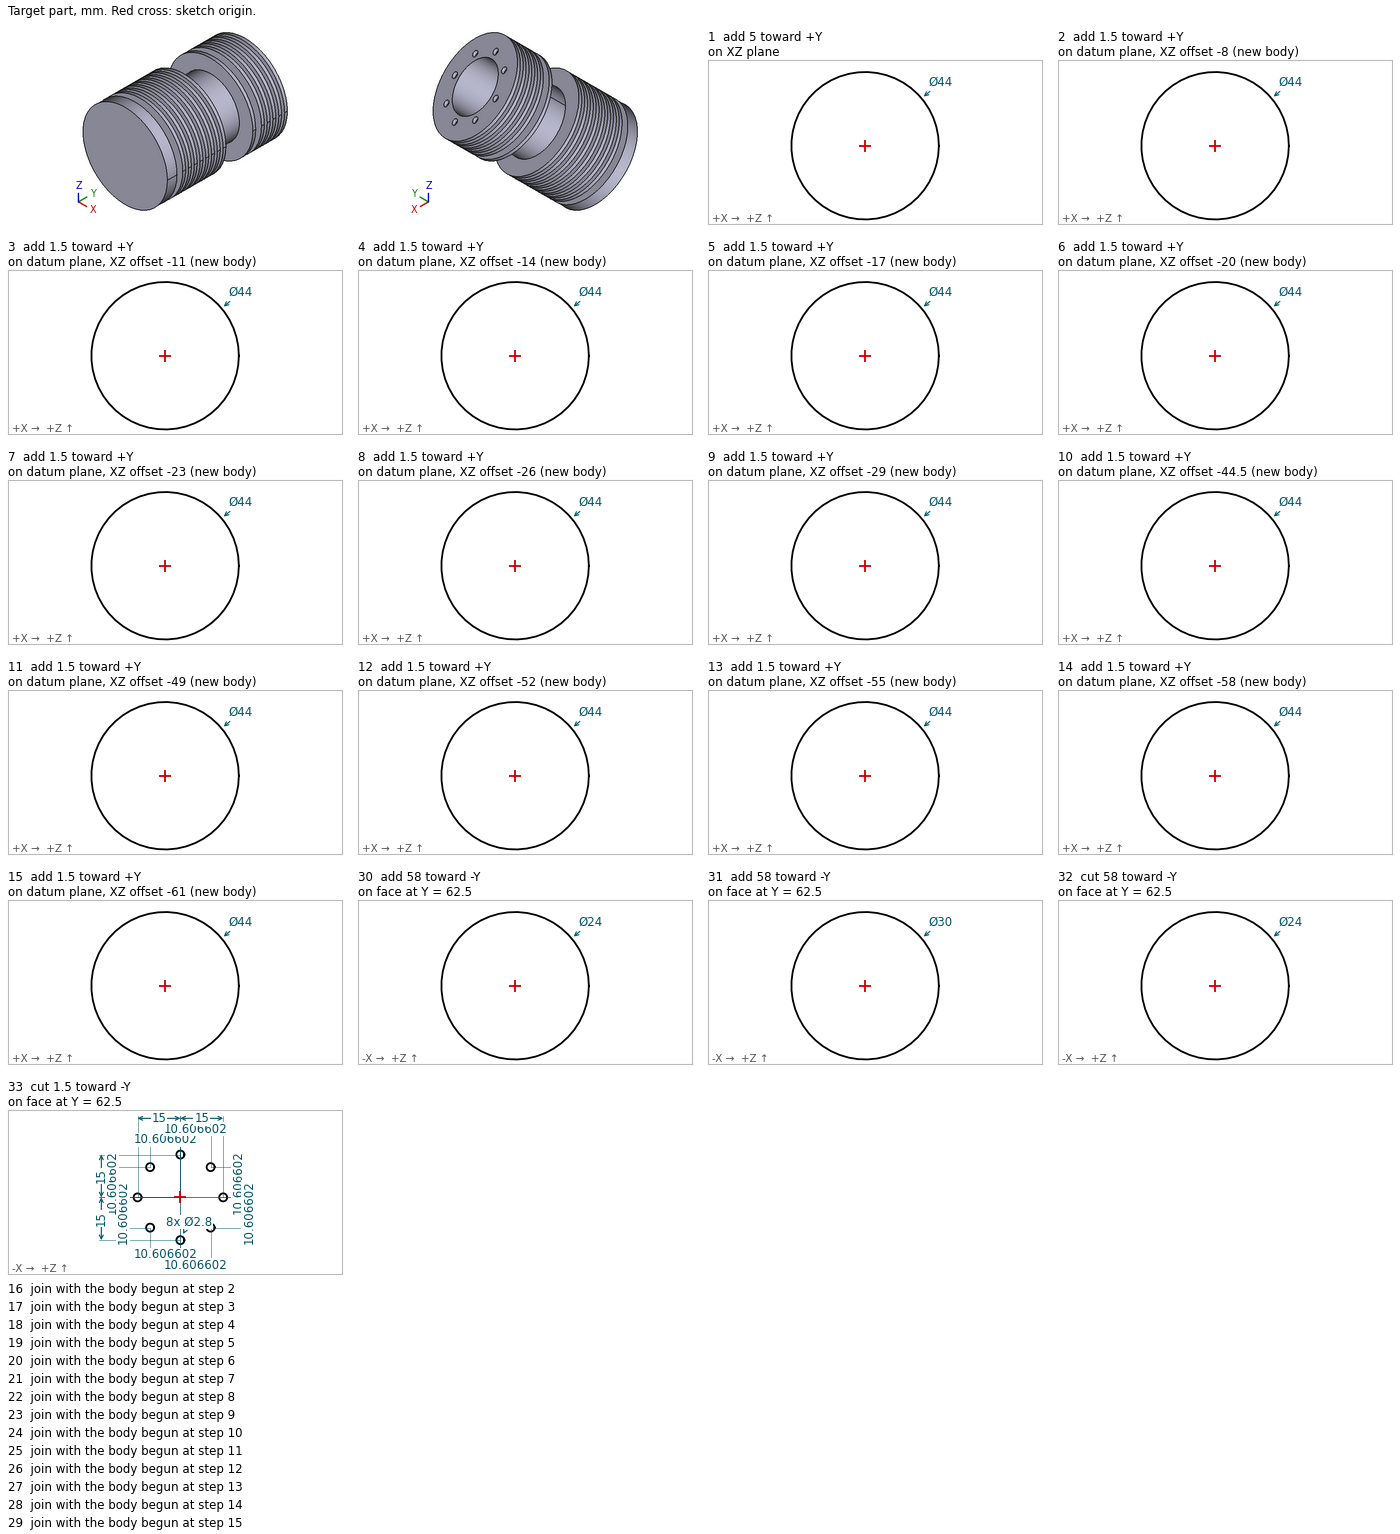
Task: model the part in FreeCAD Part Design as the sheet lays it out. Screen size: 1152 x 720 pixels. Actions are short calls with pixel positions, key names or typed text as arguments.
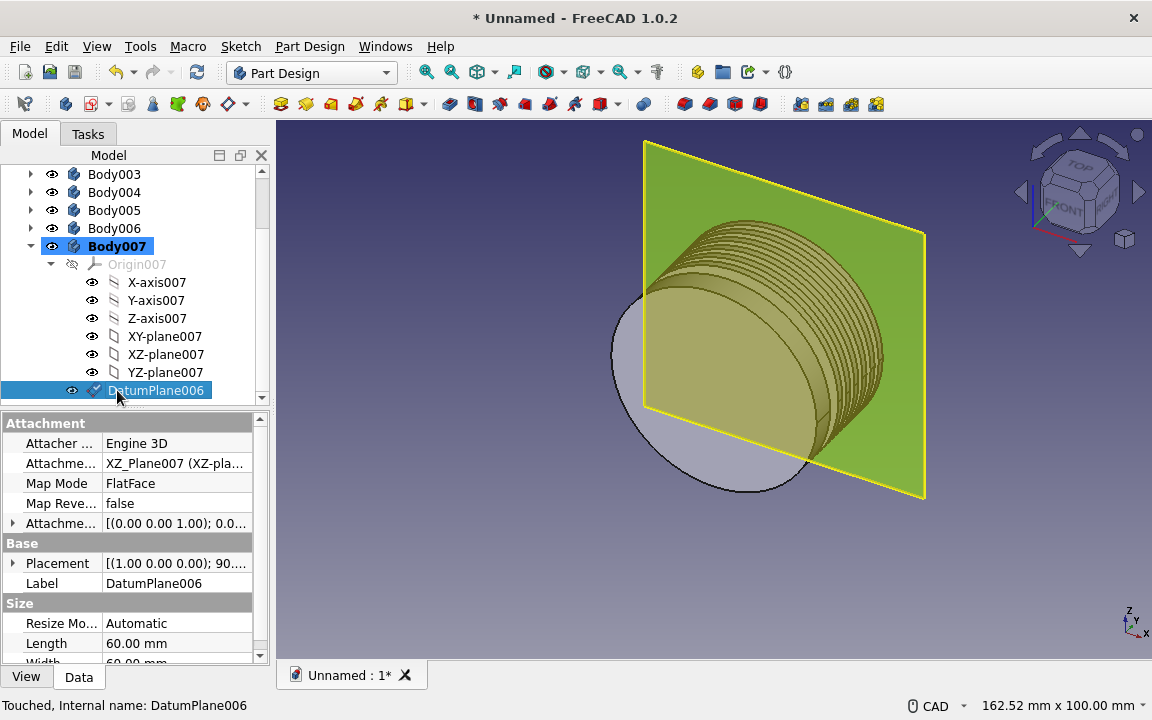
click(90, 104)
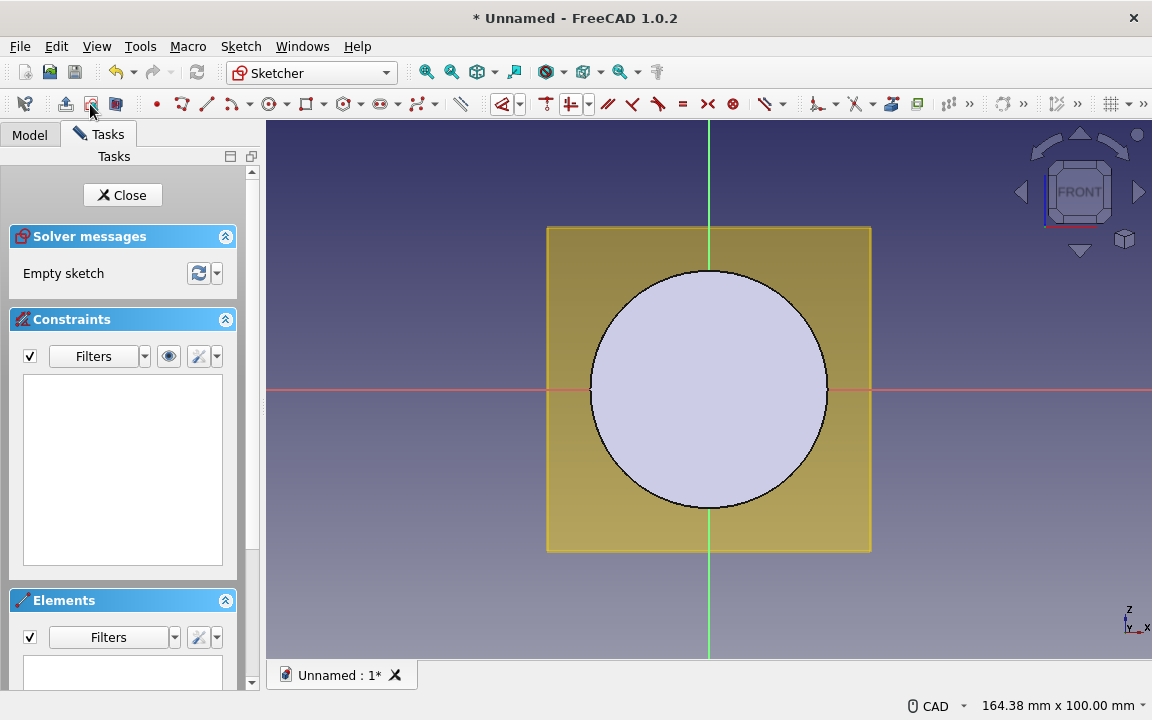
scroll(848, 390, up, 2)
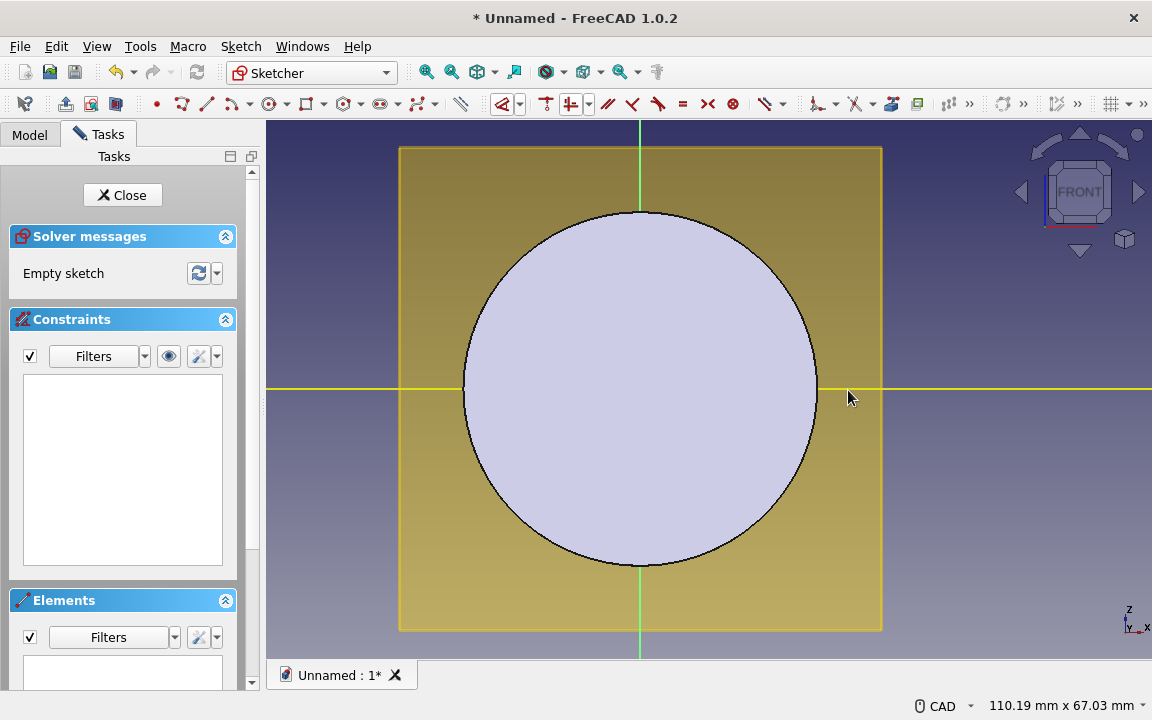
click(268, 104)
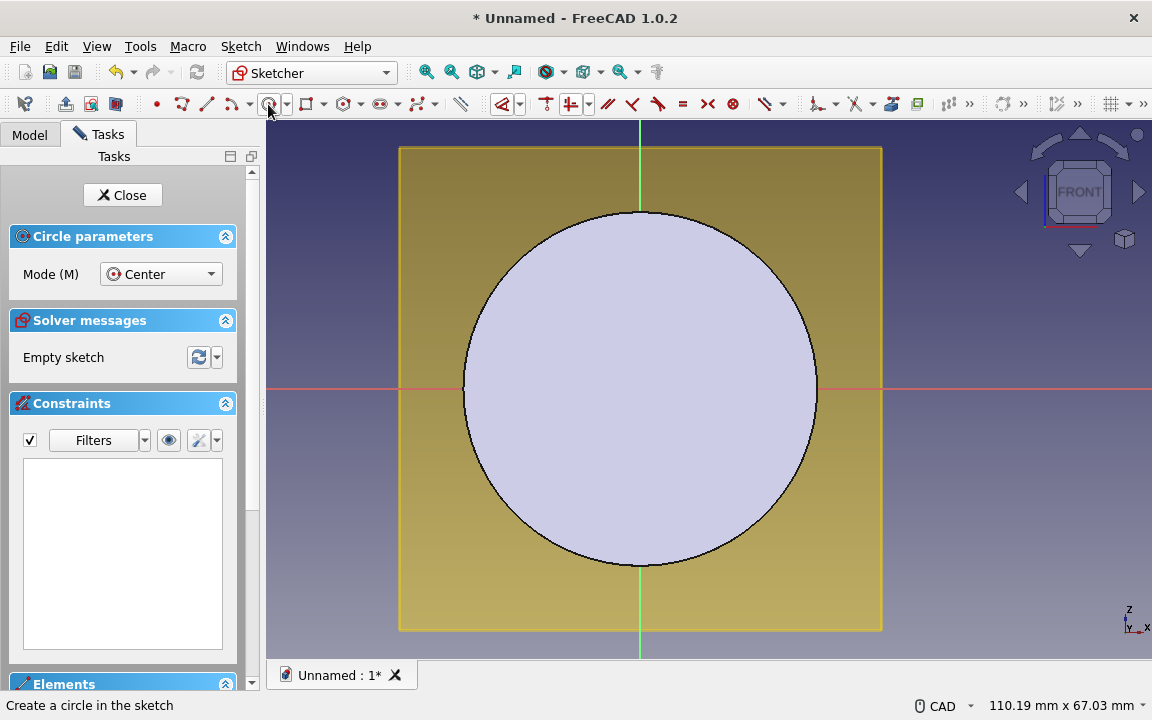
click(640, 389)
click(765, 264)
key(Escape)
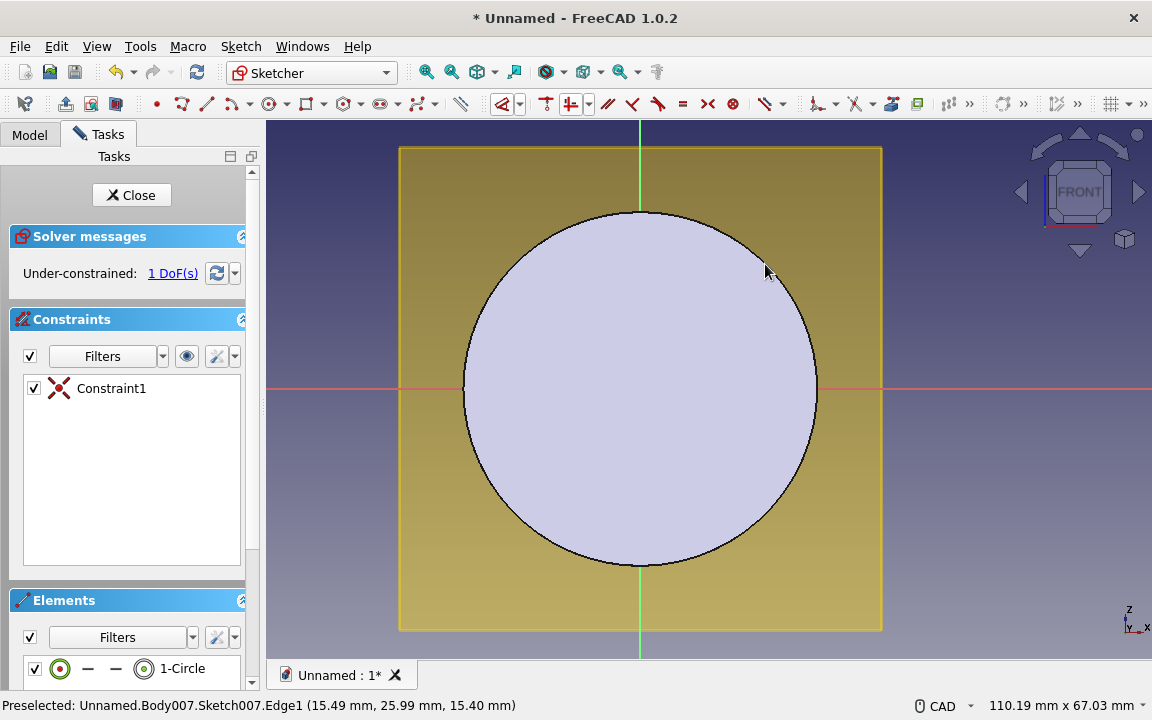
click(764, 264)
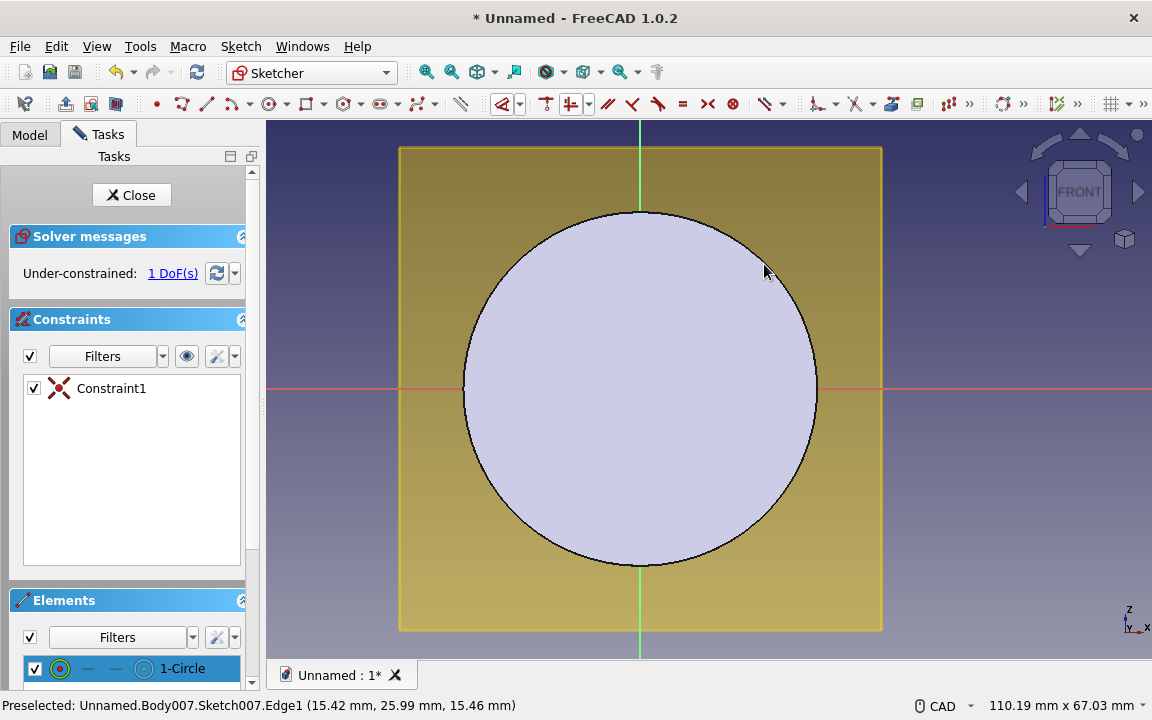
key(k)
key(o)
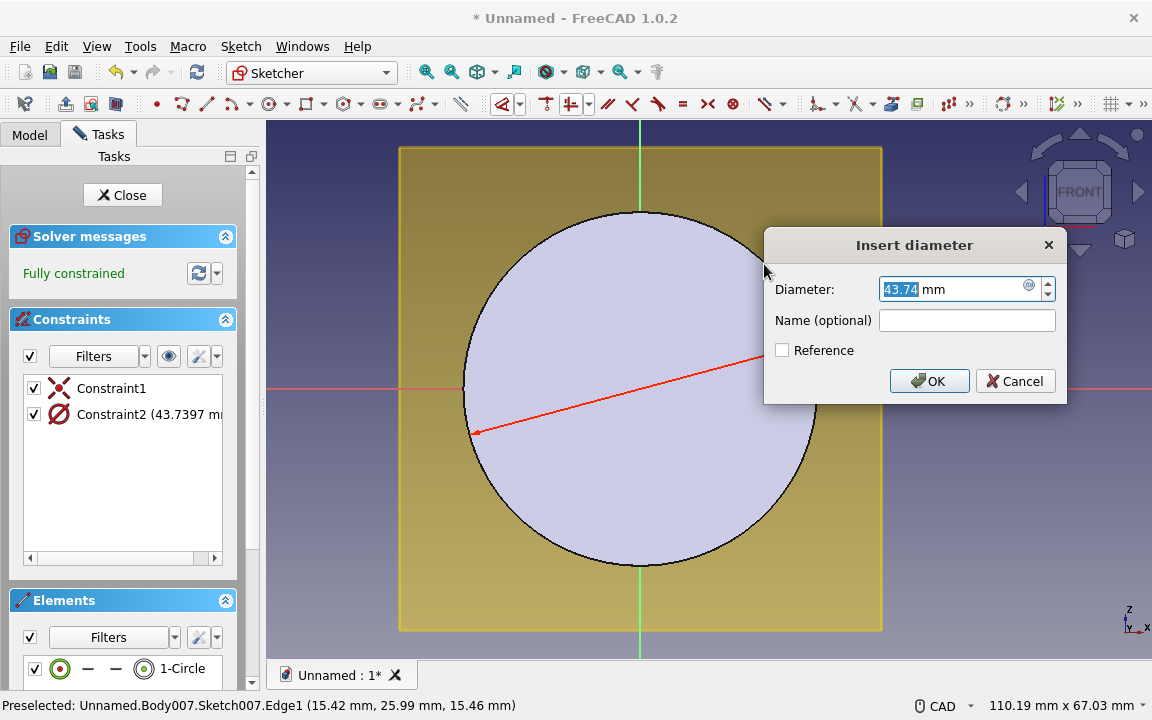
text(44)
key(Return)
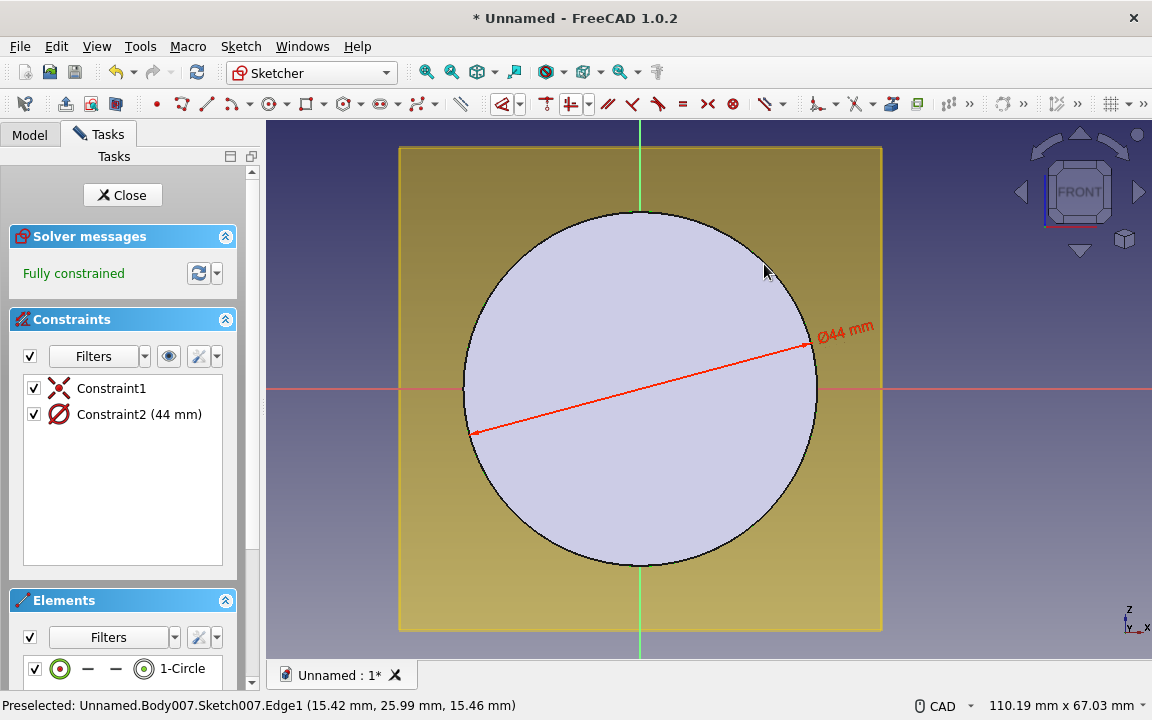
click(123, 195)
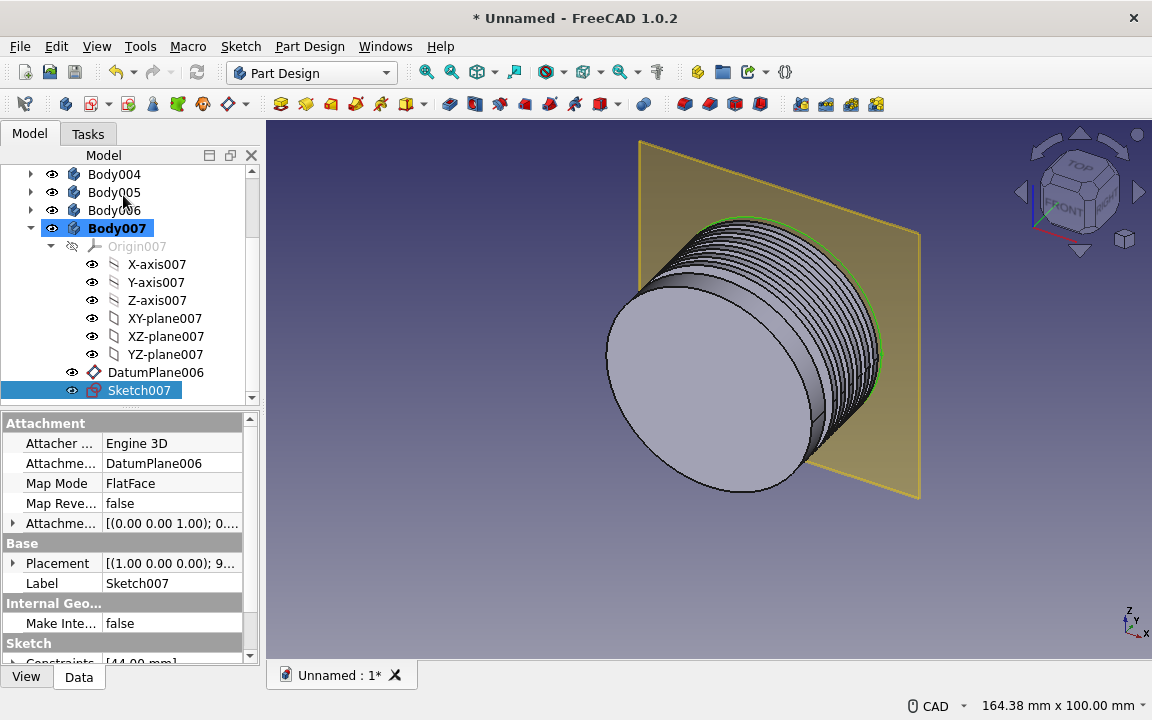
click(281, 104)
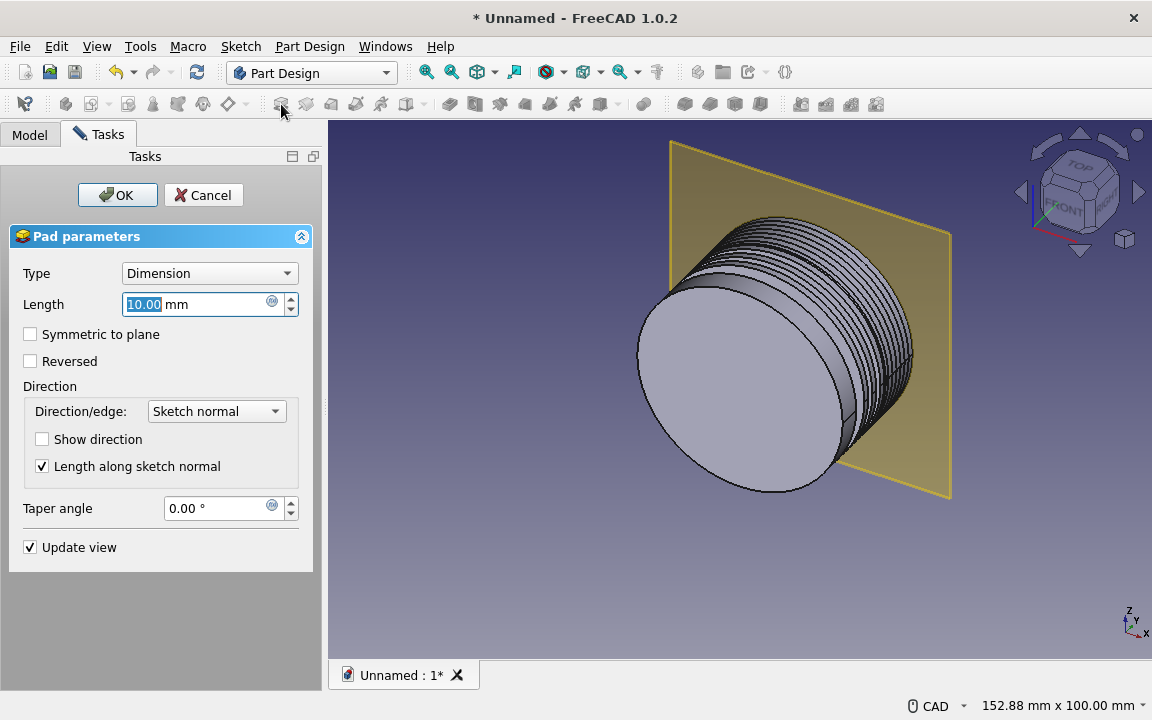
text(1.5)
key(Tab)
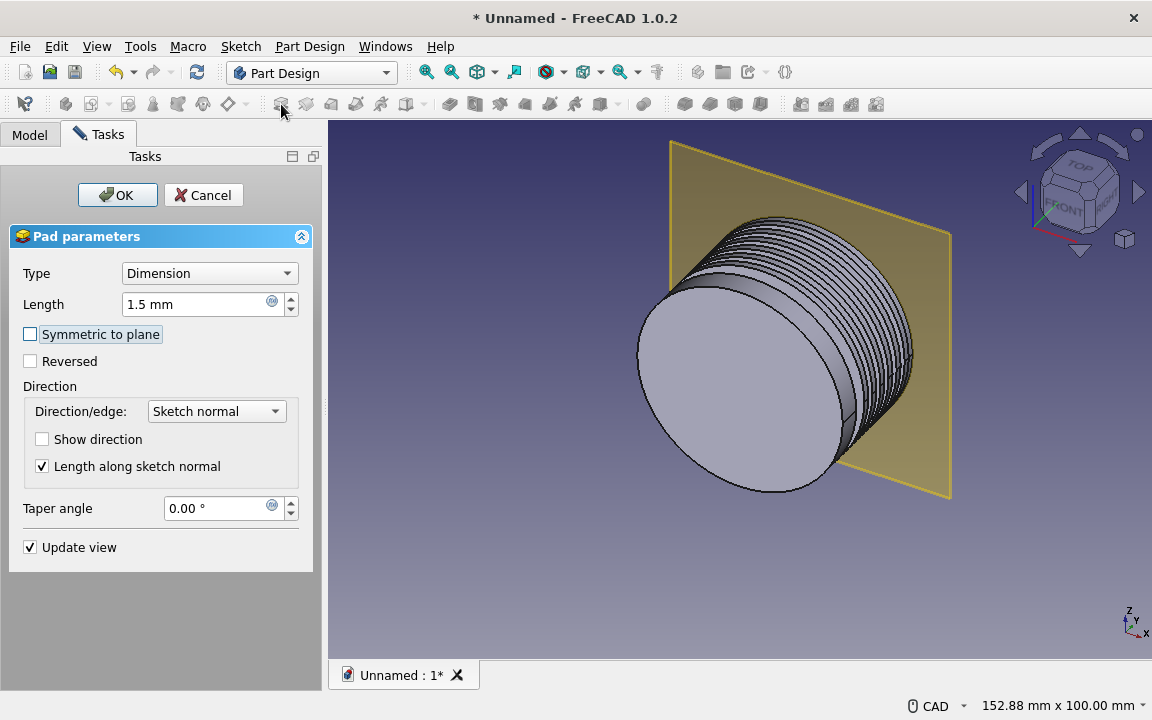
click(31, 361)